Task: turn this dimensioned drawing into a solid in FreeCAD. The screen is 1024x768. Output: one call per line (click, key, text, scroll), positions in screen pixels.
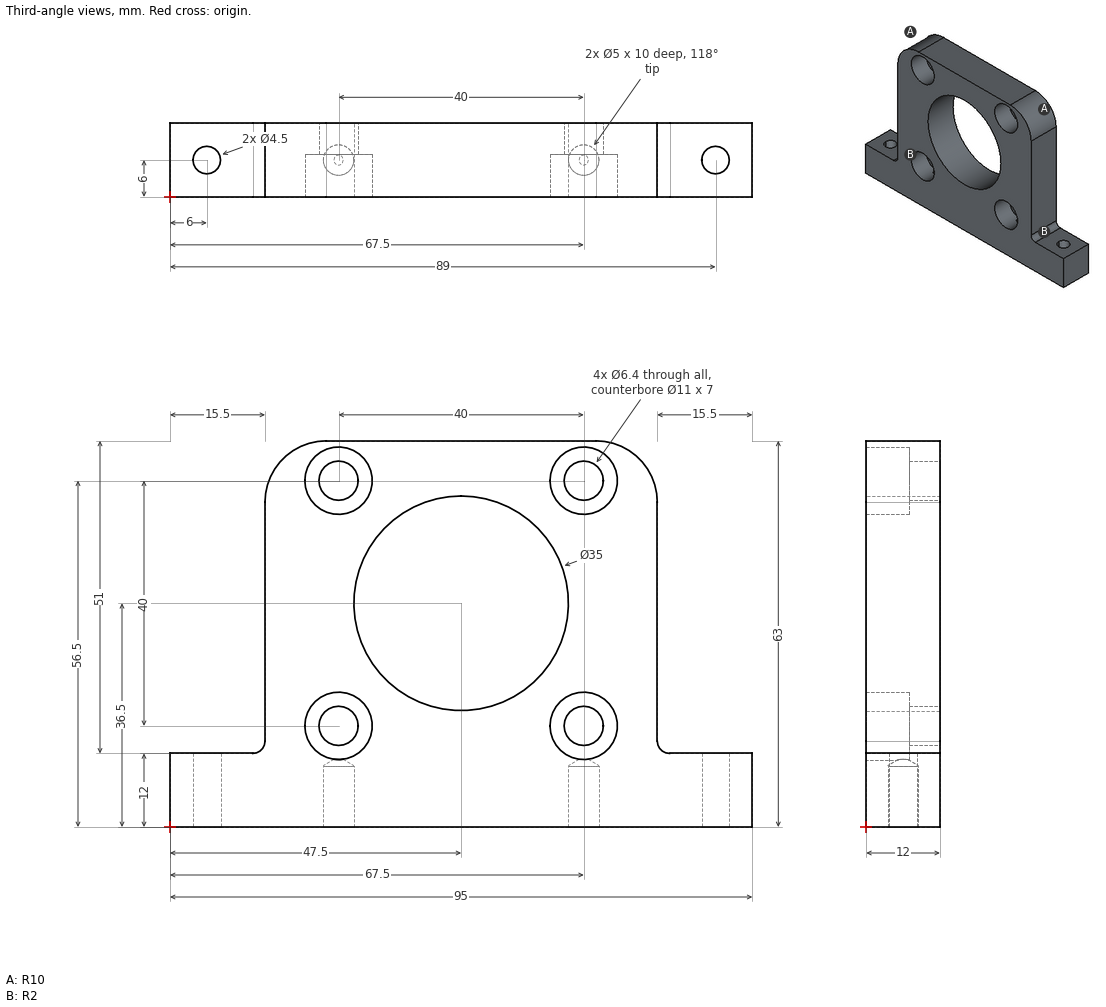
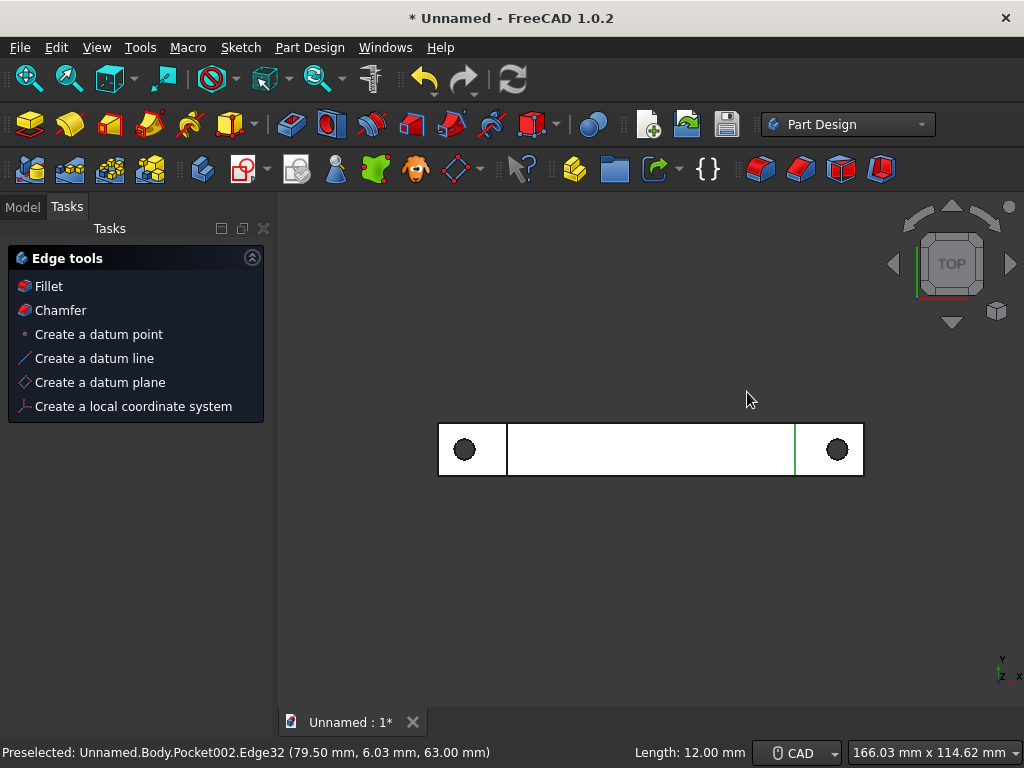
click(507, 448, ctrl)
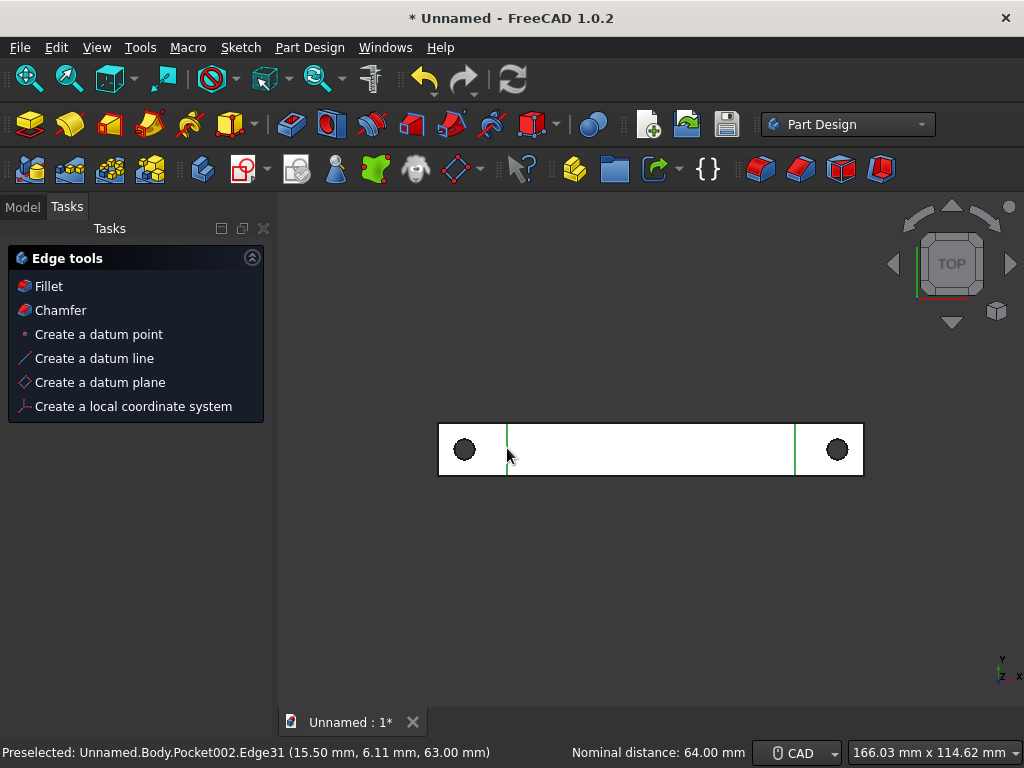
click(762, 170)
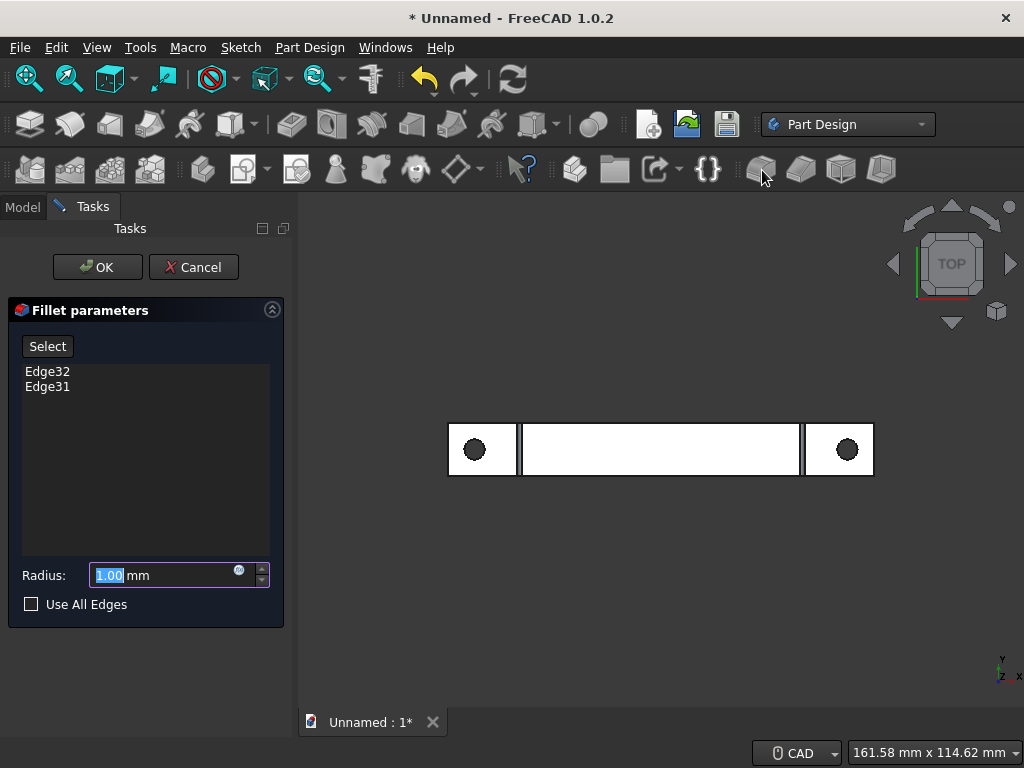
text(10)
key(Tab)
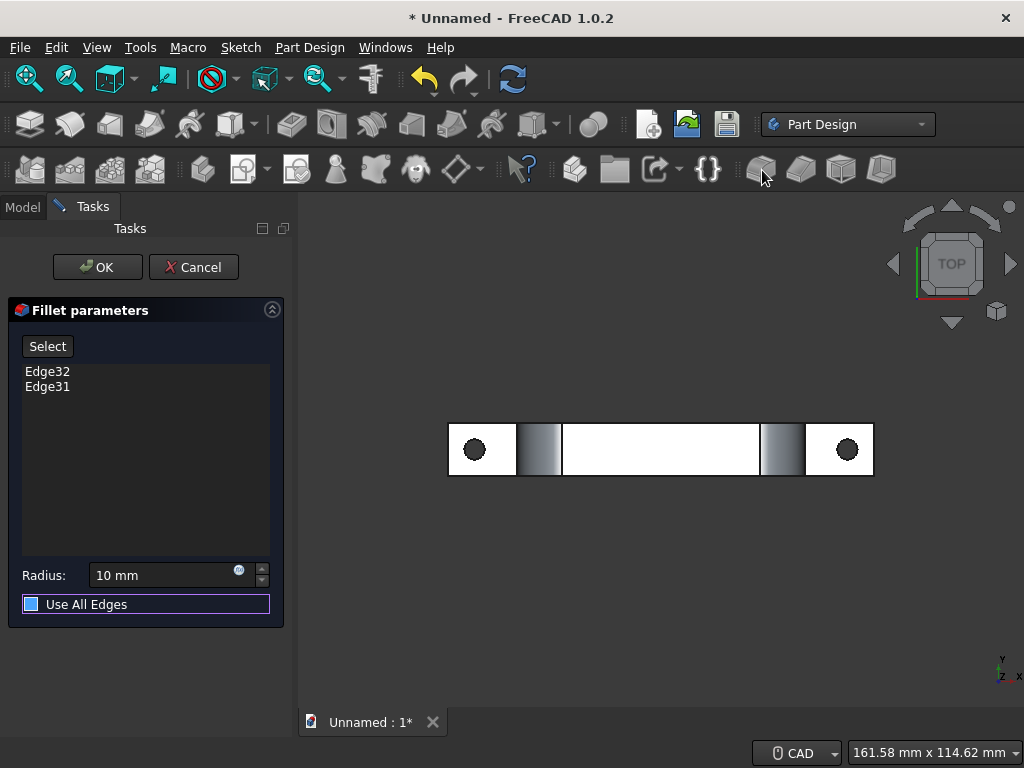
click(98, 267)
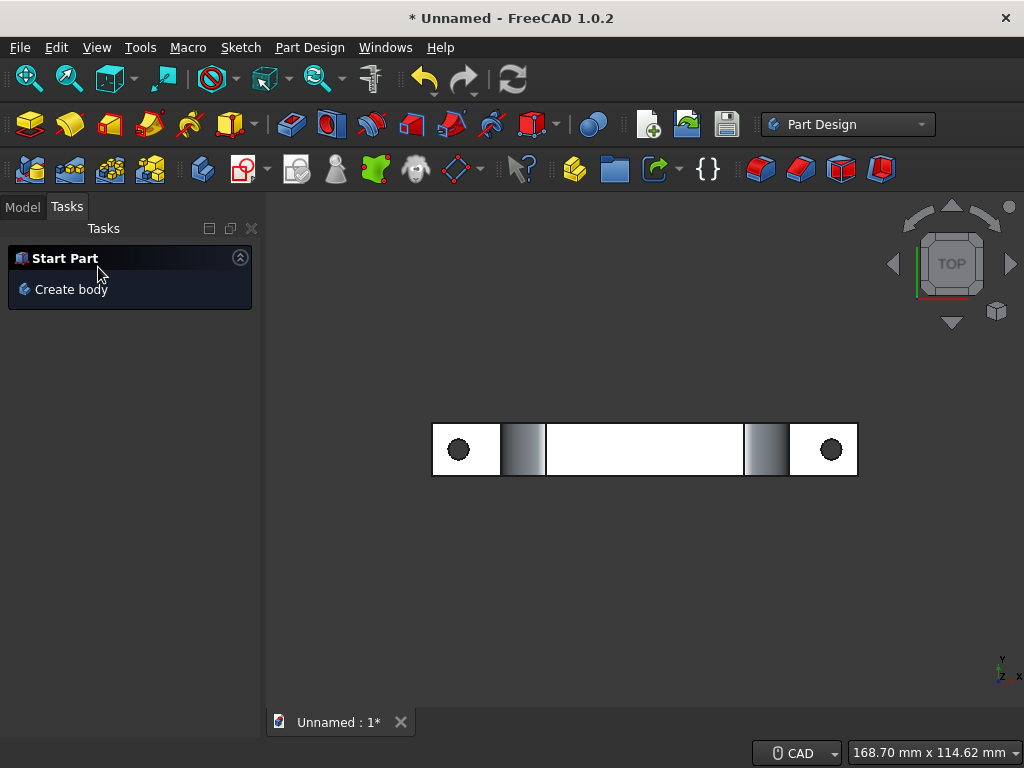
click(244, 170)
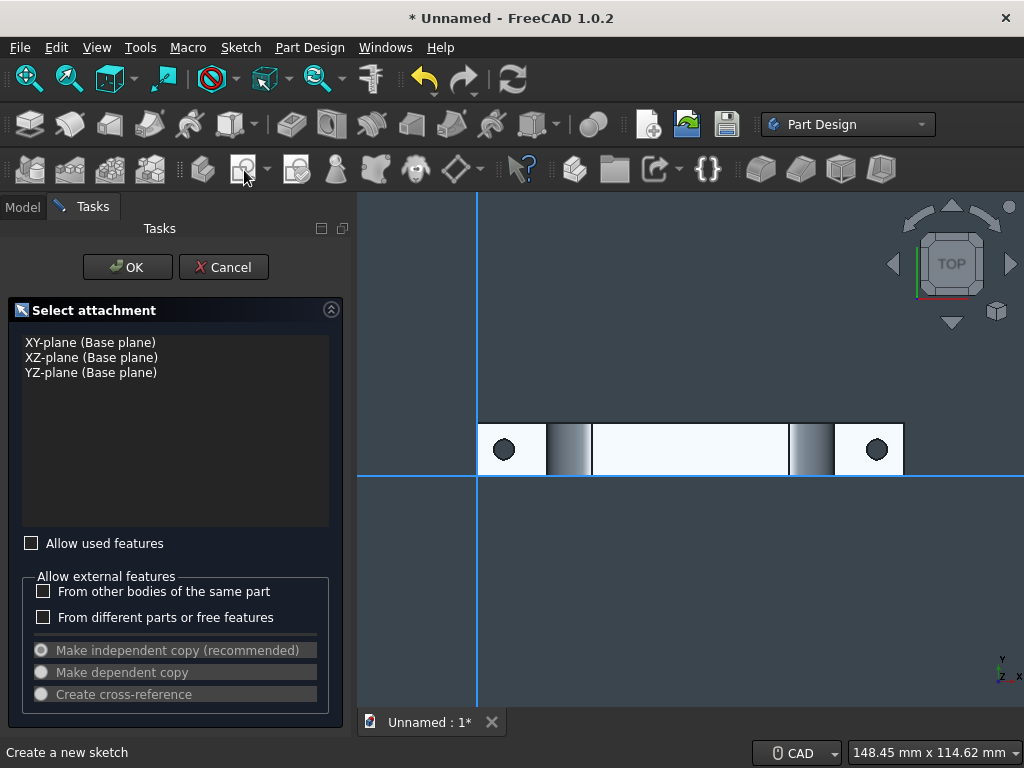
click(82, 342)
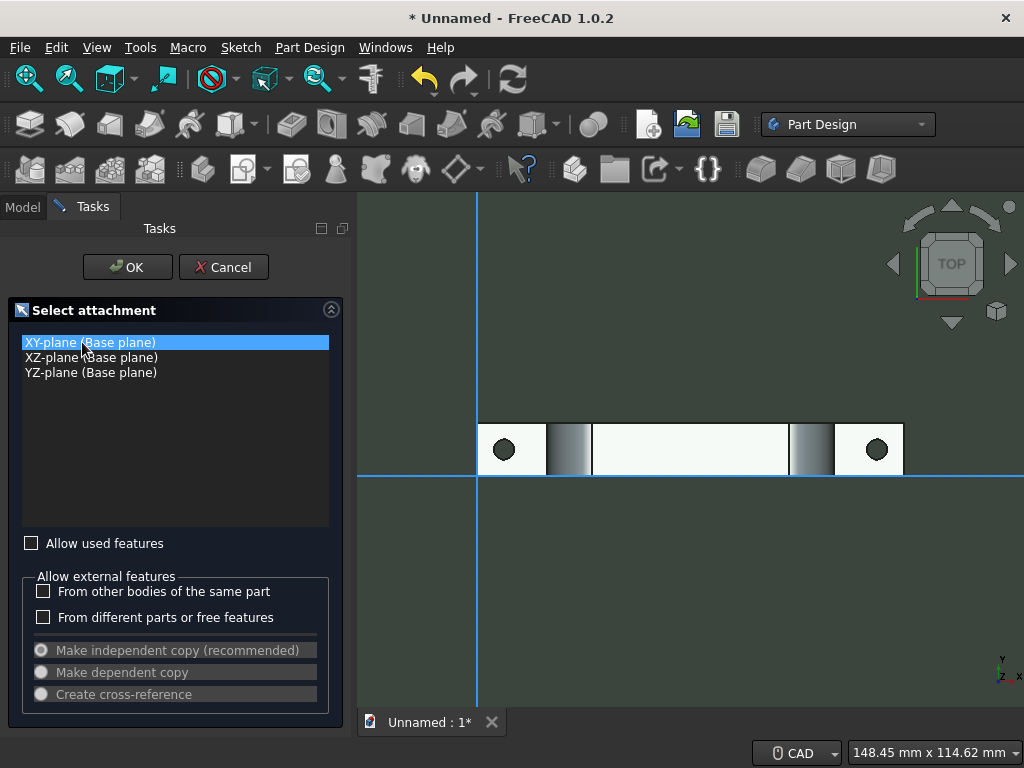
click(128, 267)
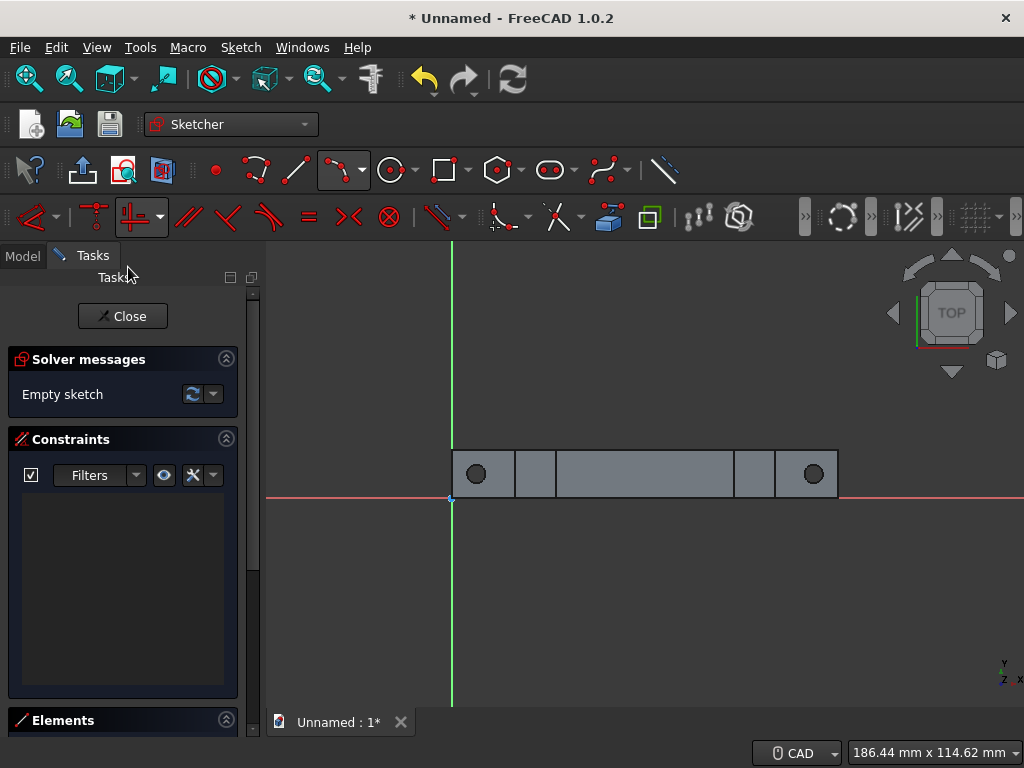
click(164, 170)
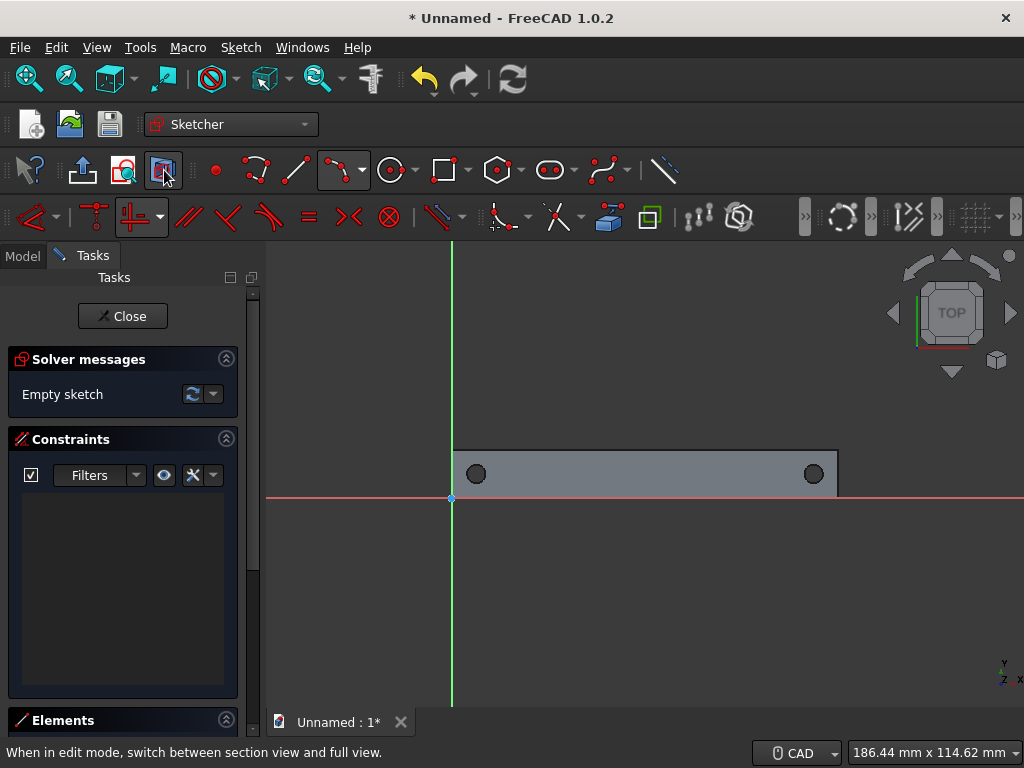
scroll(630, 496, up, 2)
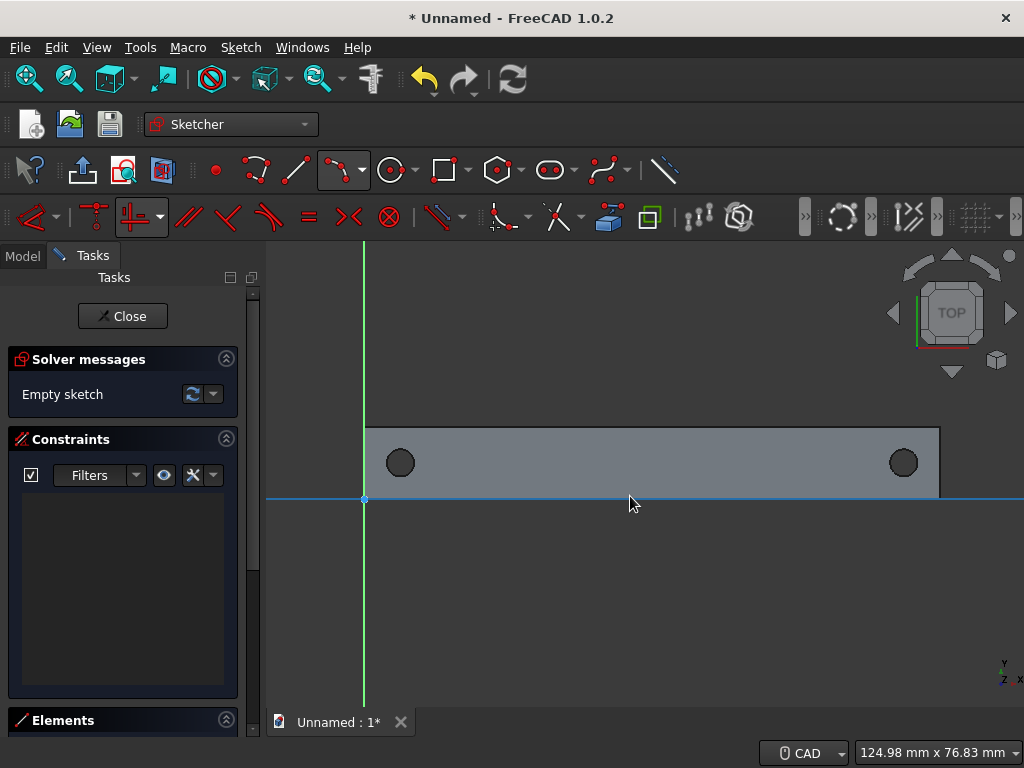
click(392, 170)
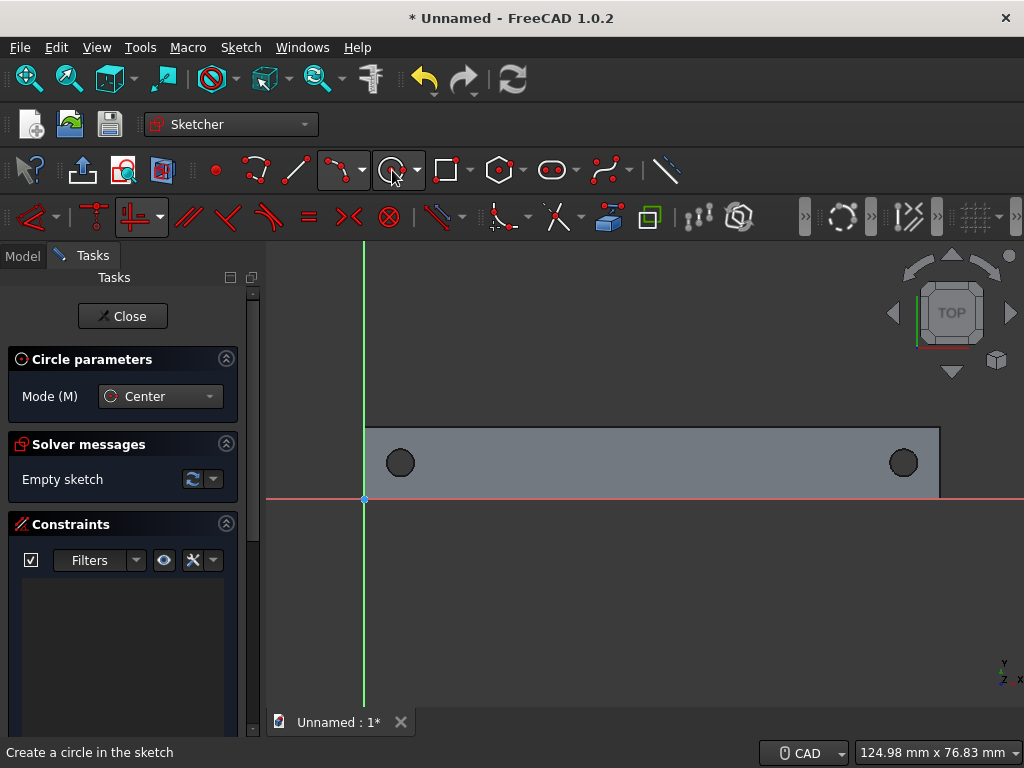
scroll(773, 463, up, 3)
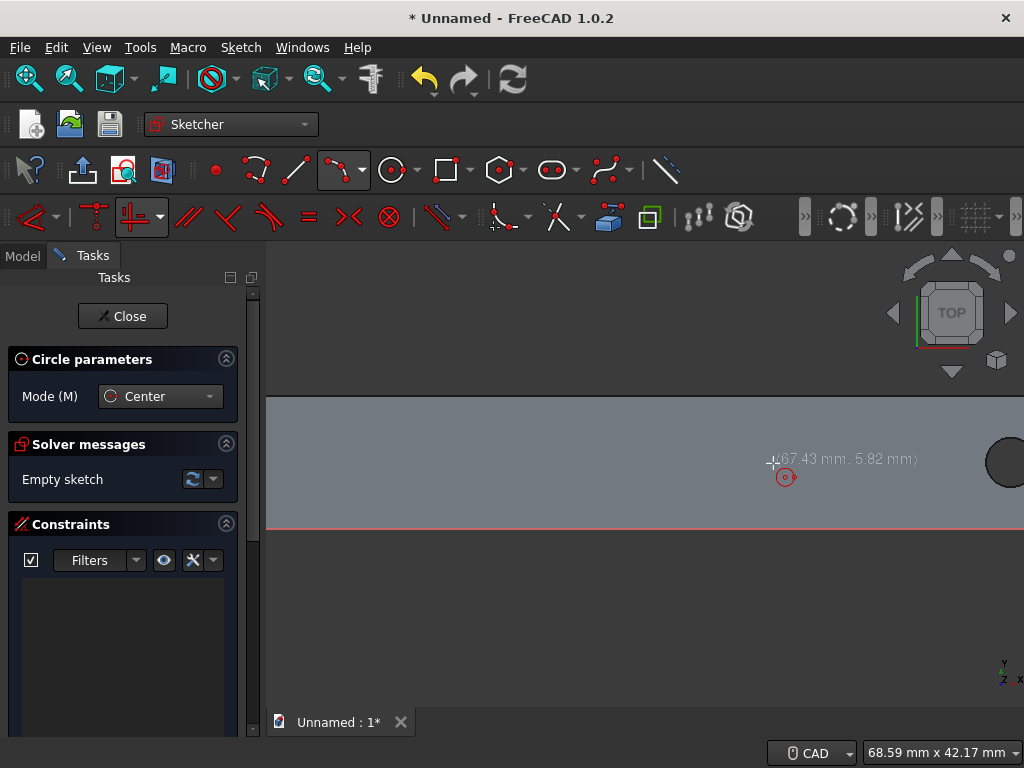
click(773, 462)
click(793, 443)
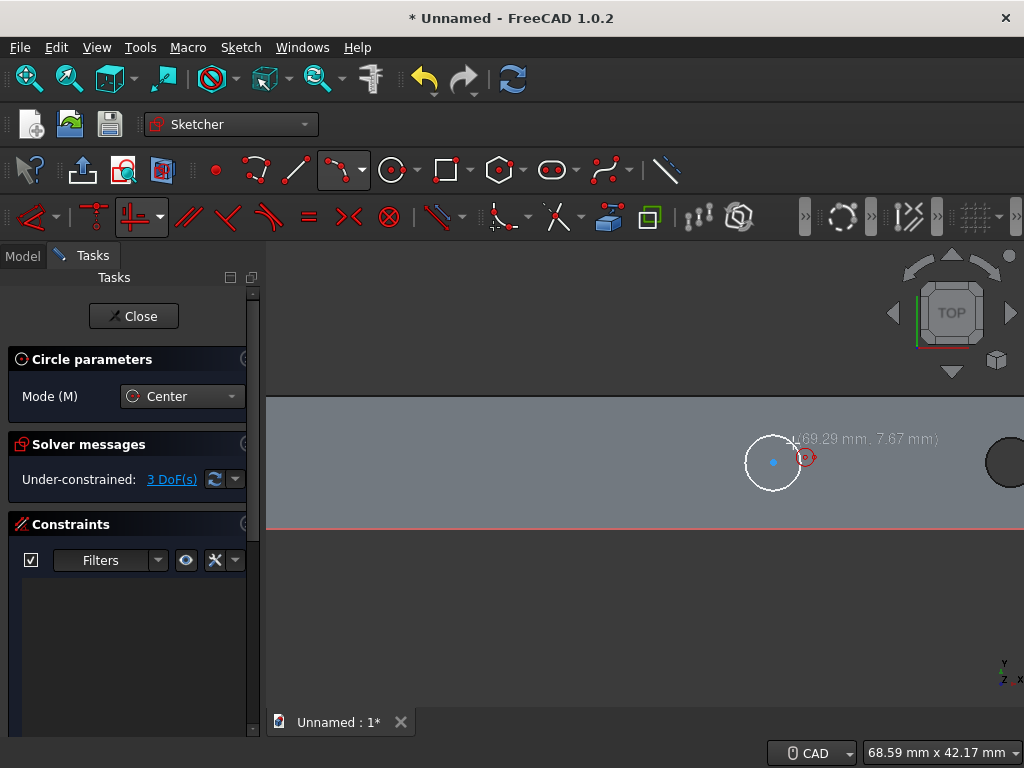
click(331, 462)
click(351, 443)
key(Escape)